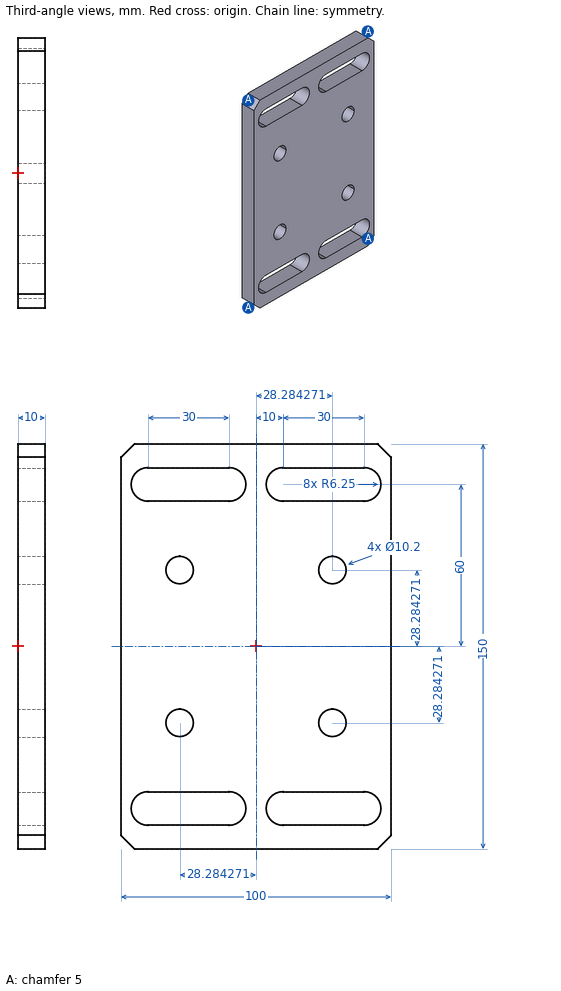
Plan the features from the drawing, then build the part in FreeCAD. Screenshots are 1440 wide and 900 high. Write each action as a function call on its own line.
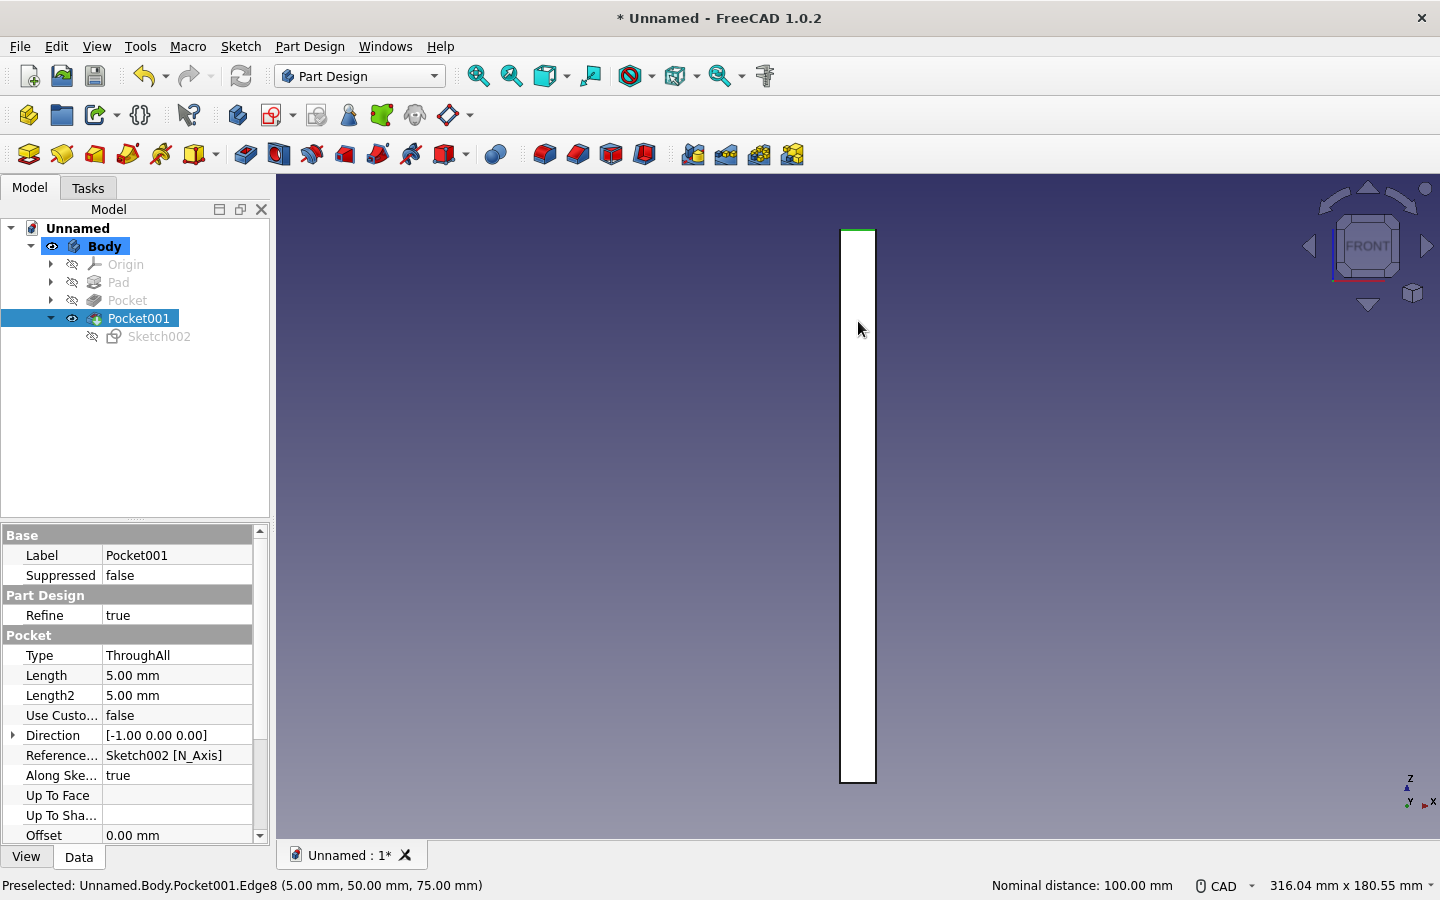
click(858, 782, ctrl)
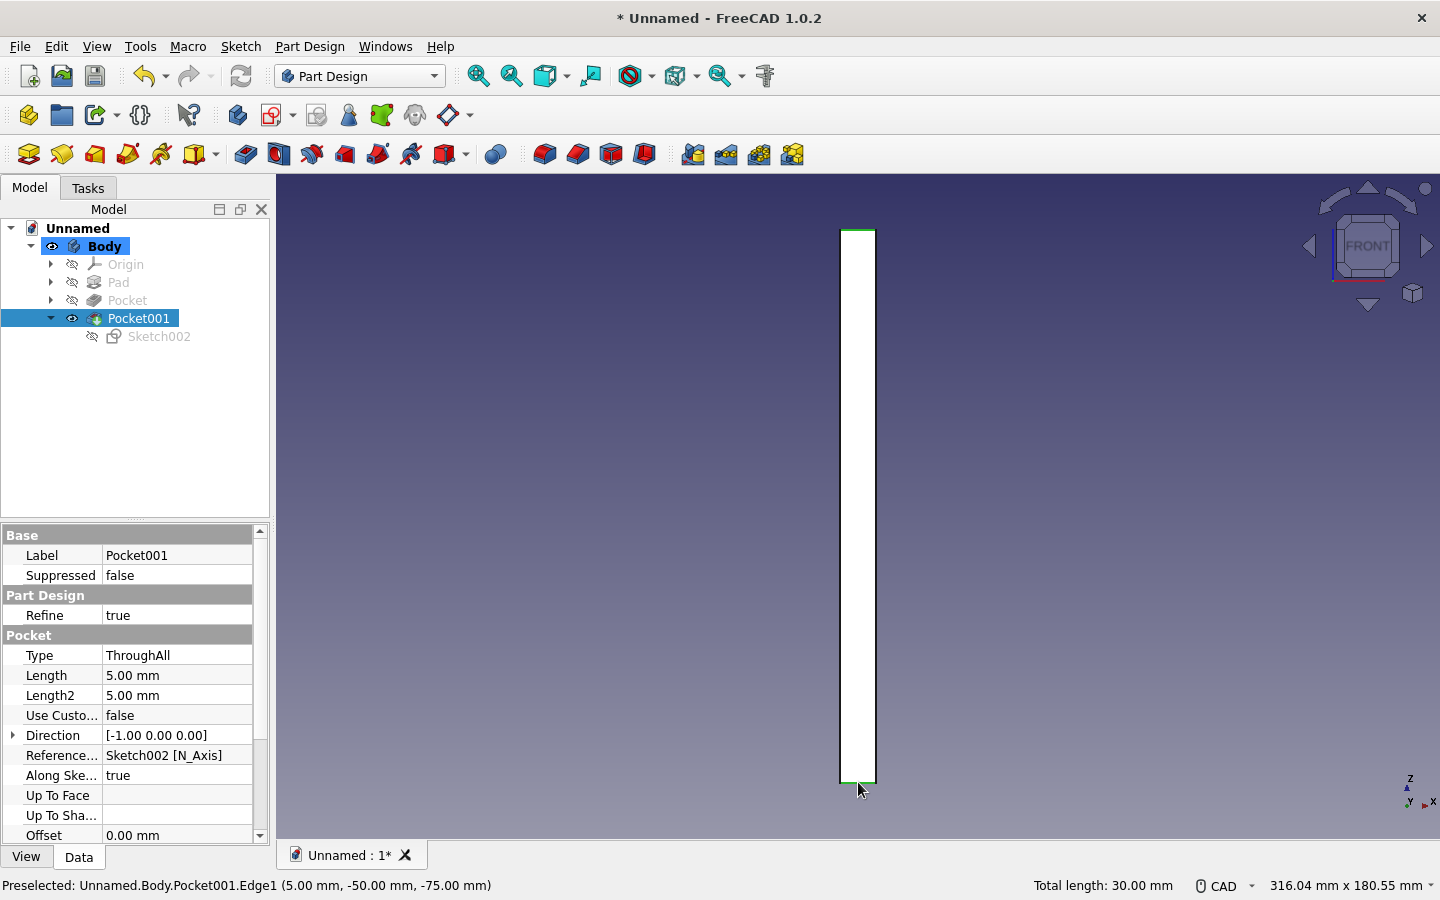
key(3)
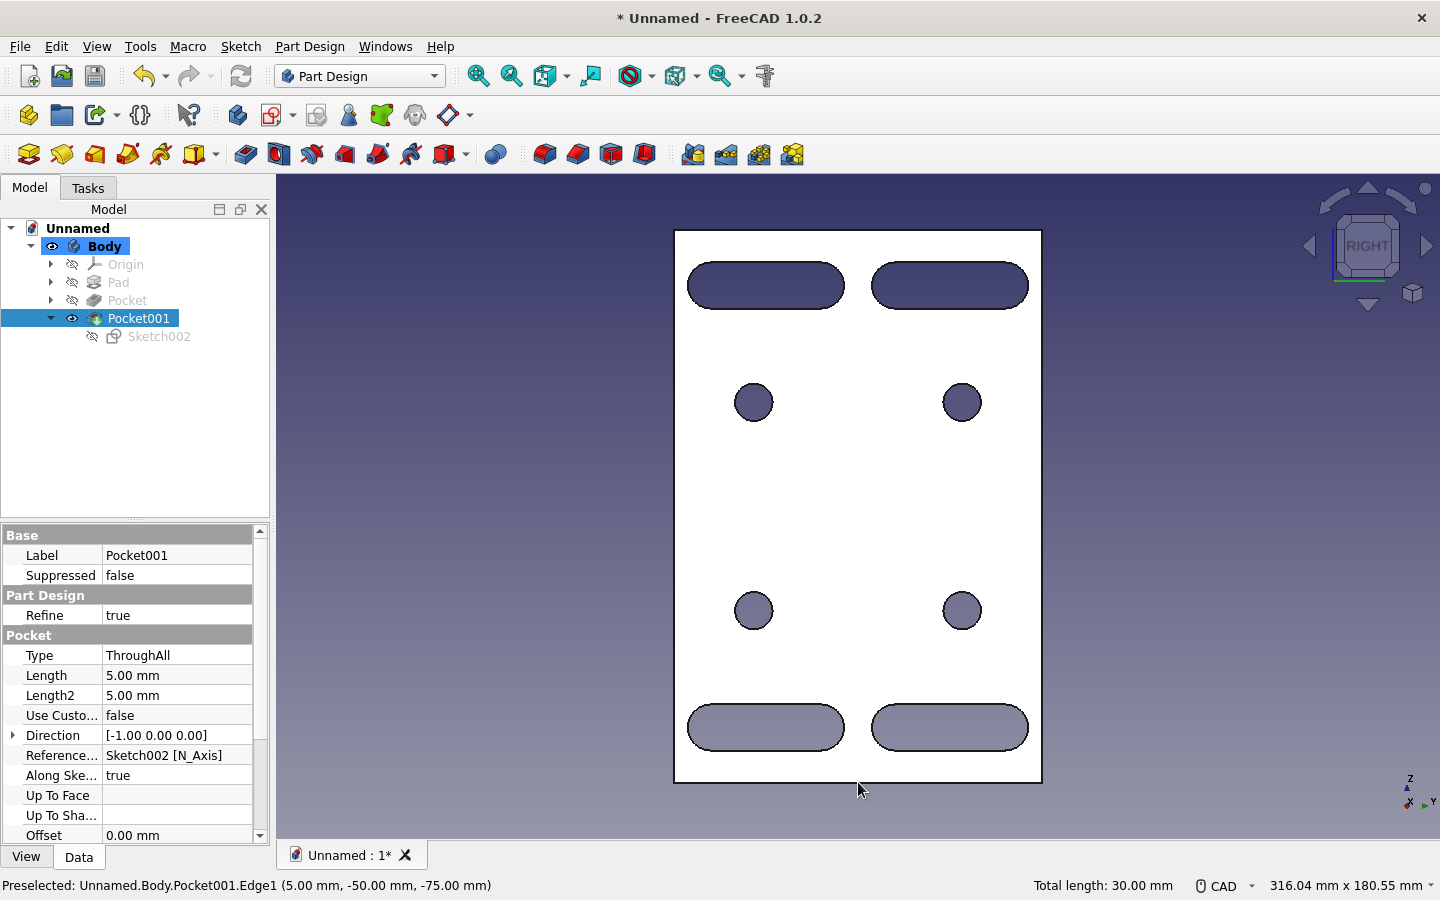
key(5)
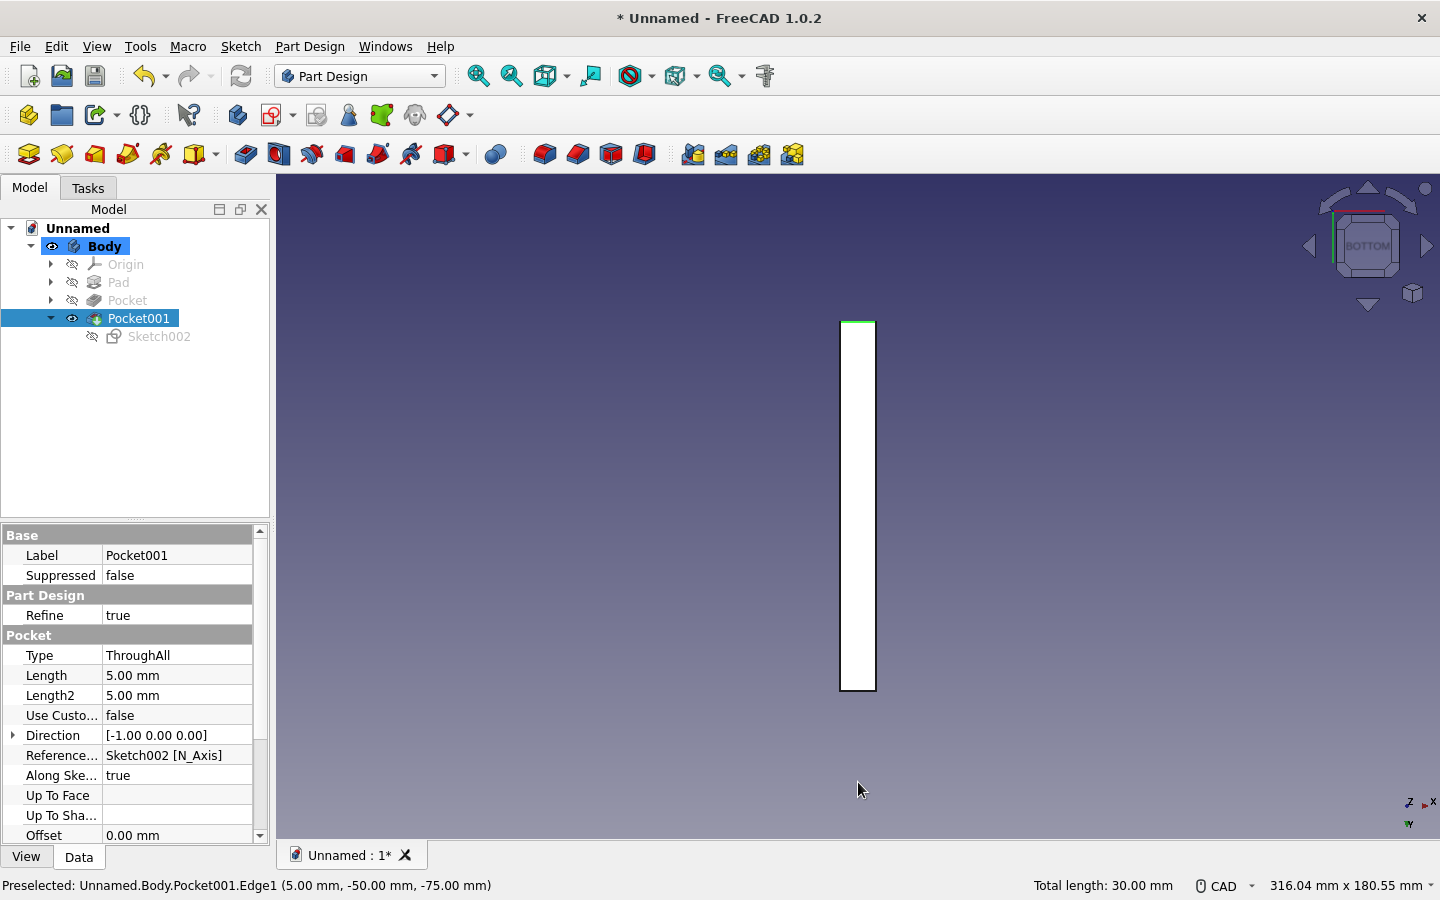
click(858, 690, ctrl)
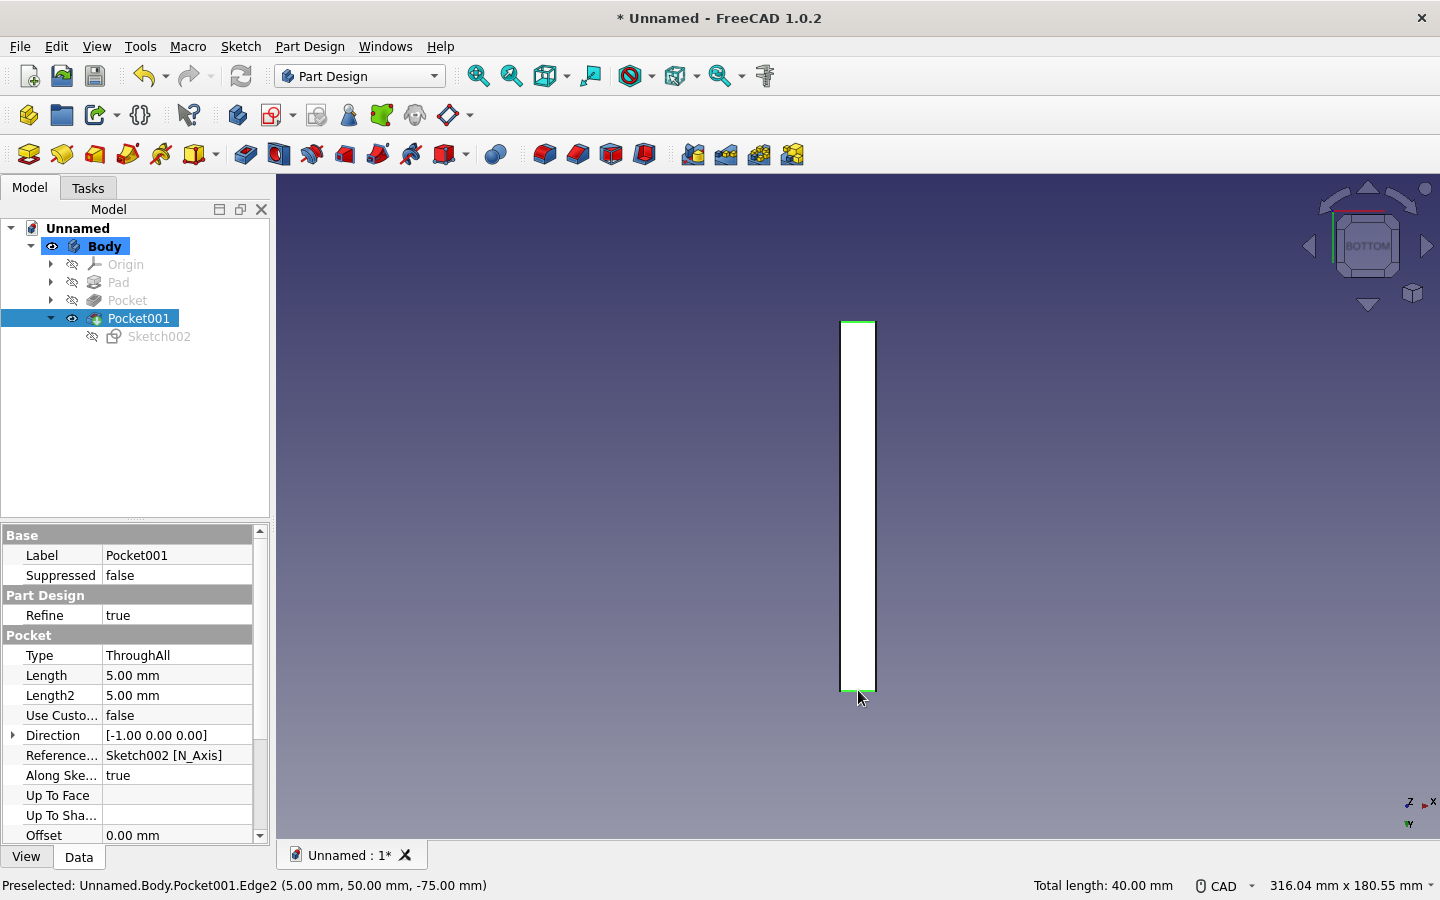
click(578, 154)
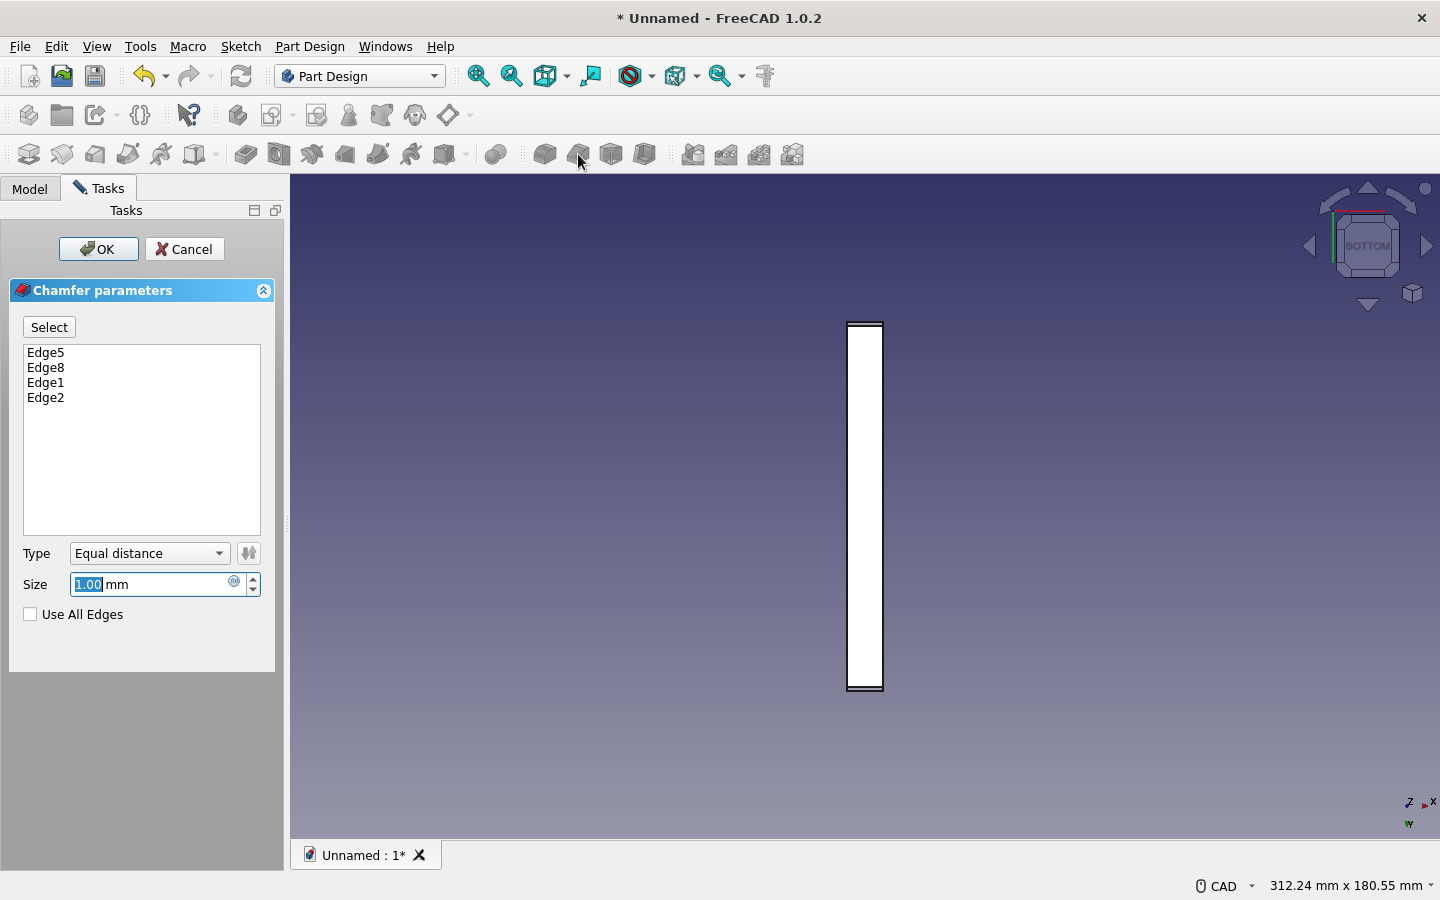
text(5)
key(Tab)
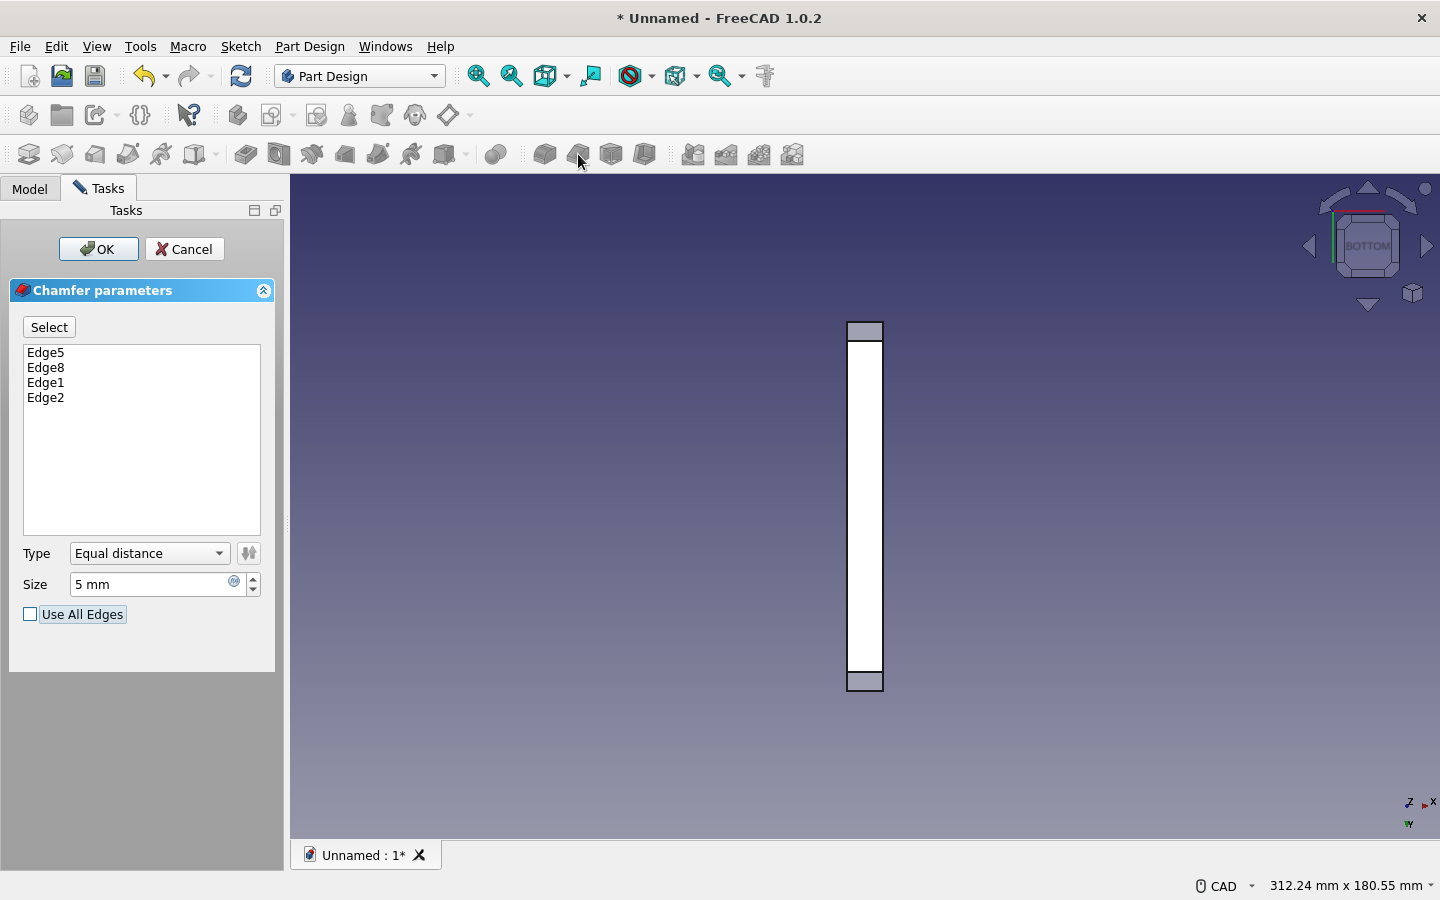
click(99, 249)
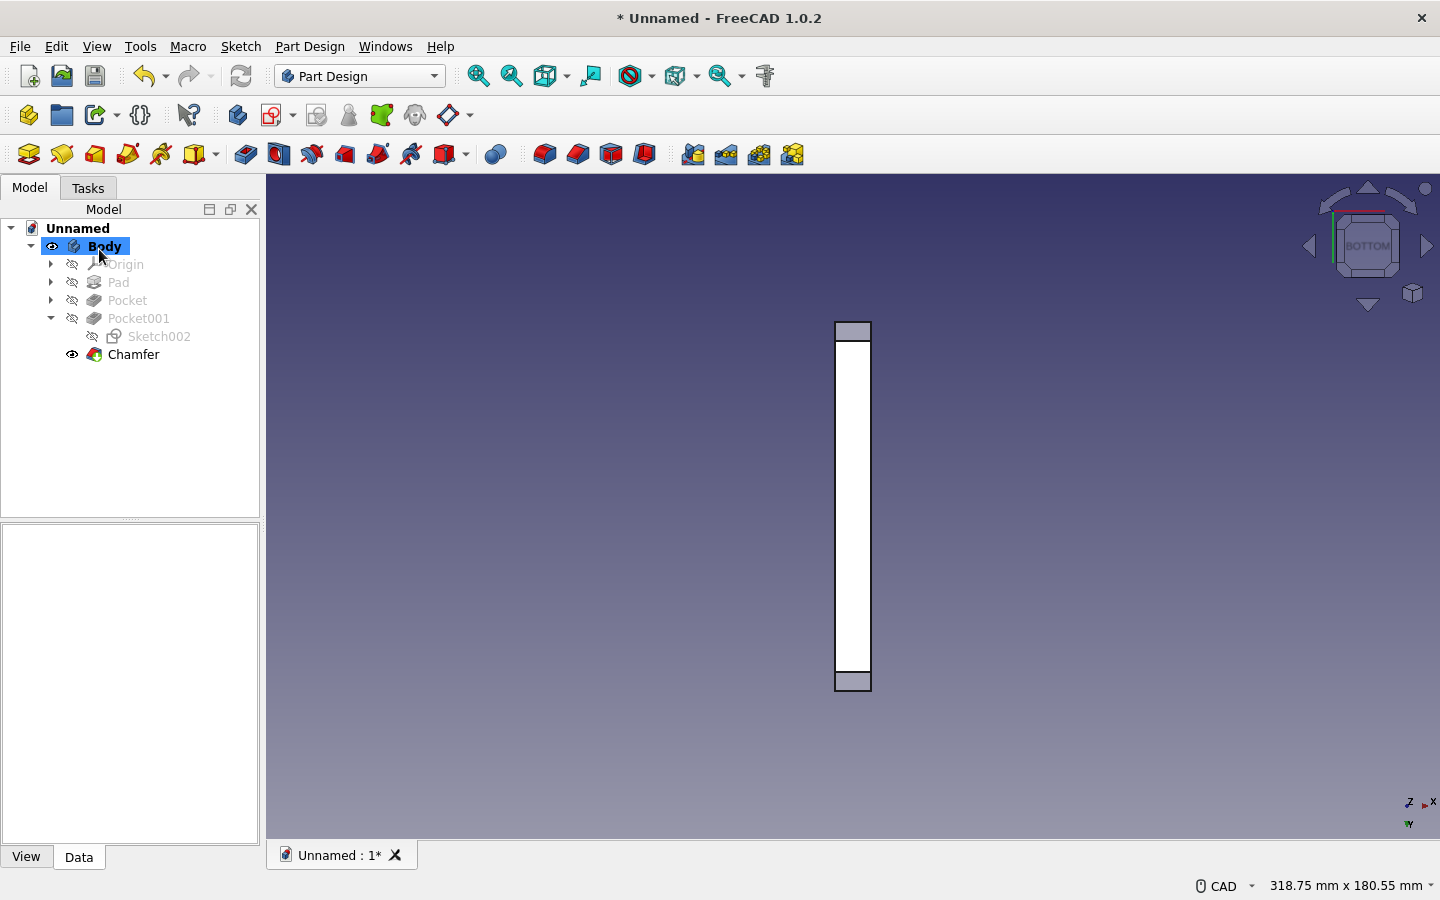
key(0)